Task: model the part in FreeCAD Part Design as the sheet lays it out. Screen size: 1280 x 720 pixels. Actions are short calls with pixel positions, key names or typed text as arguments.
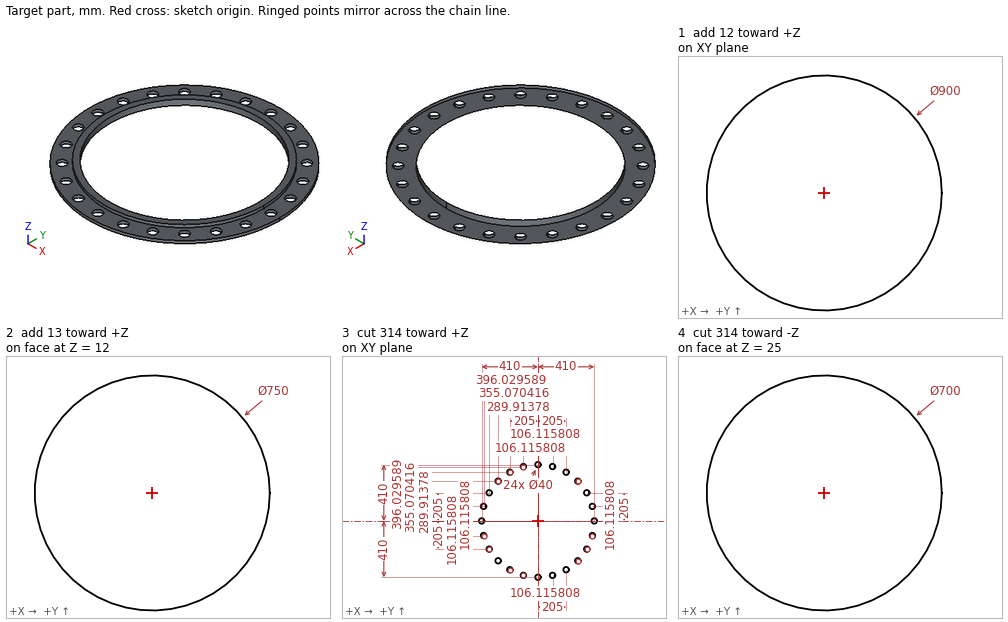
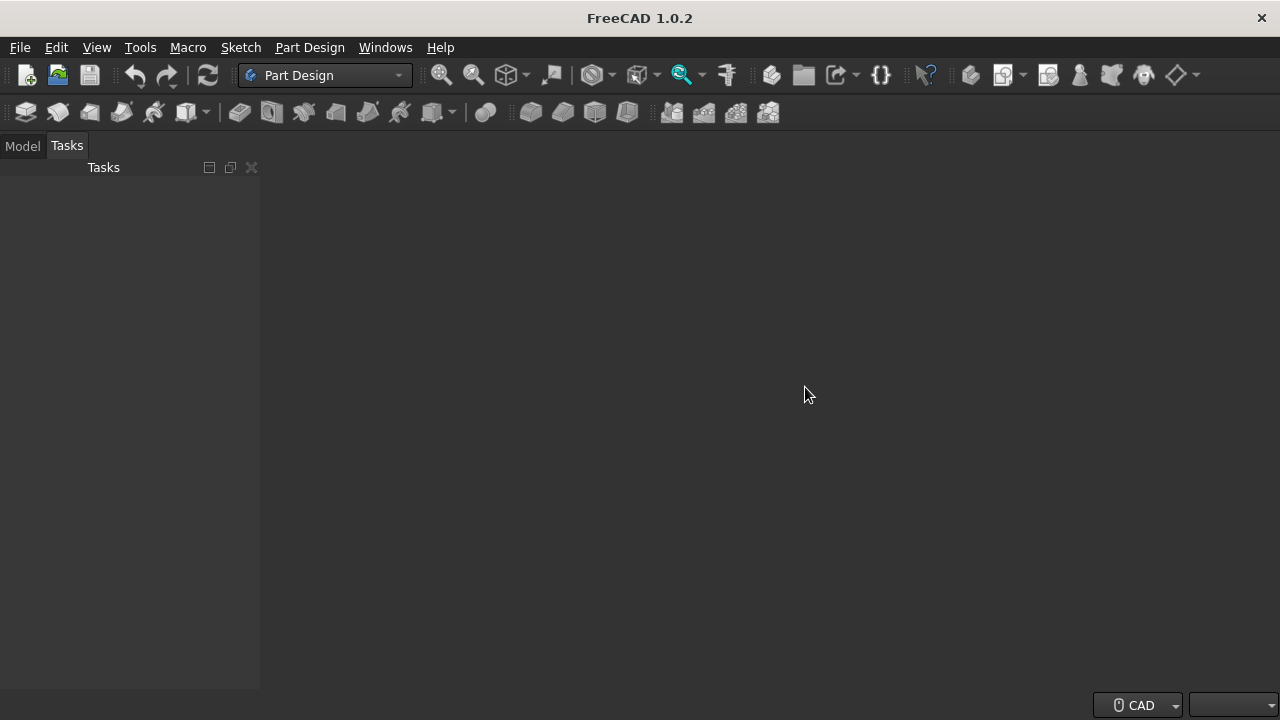
click(26, 76)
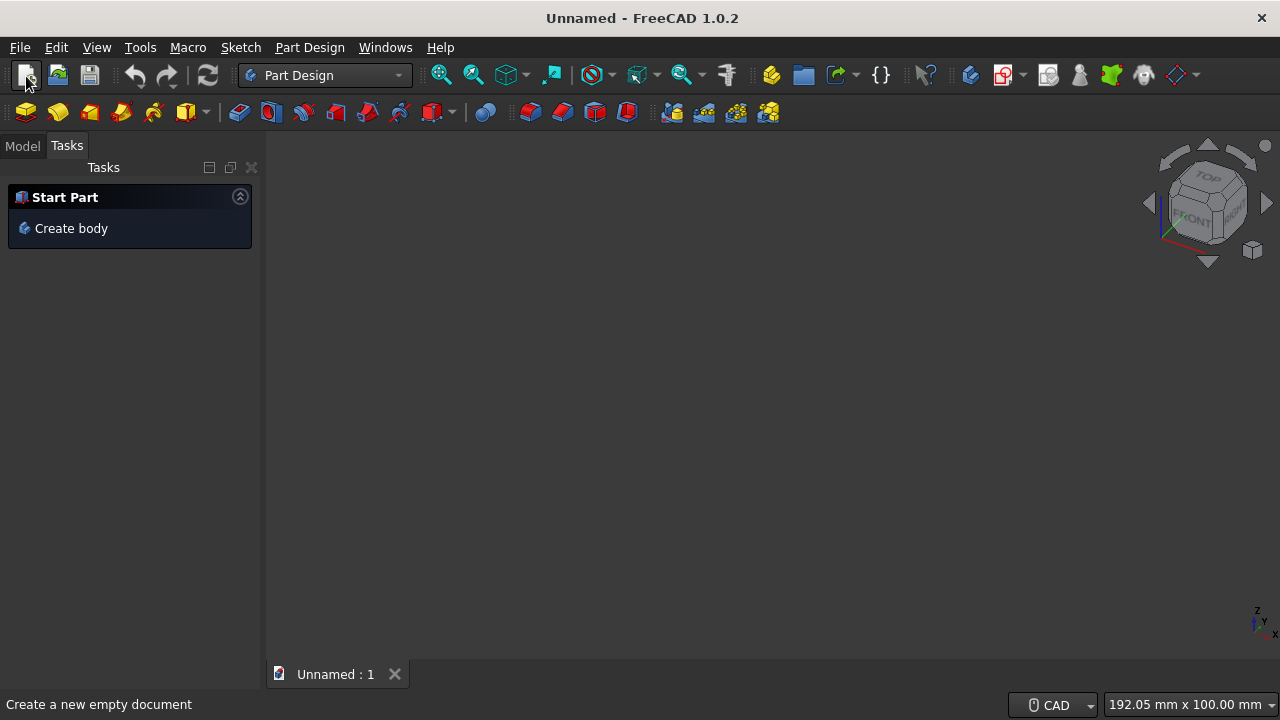
click(1004, 76)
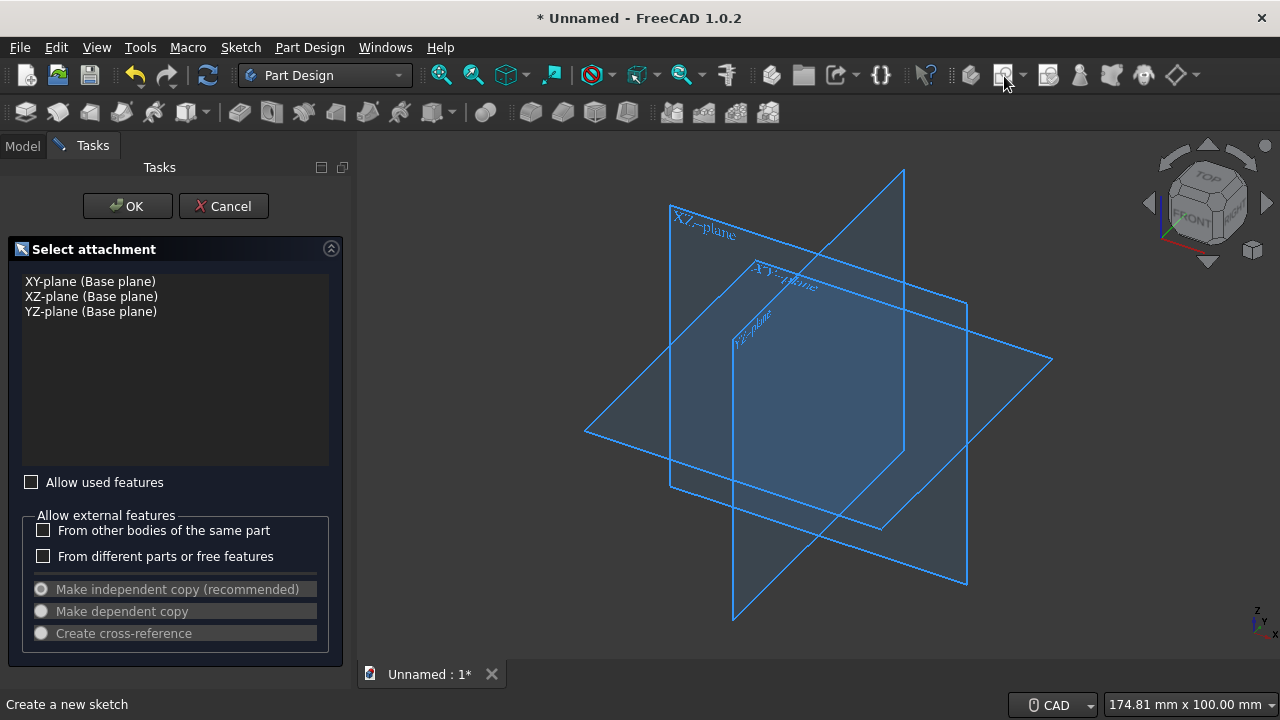
click(82, 282)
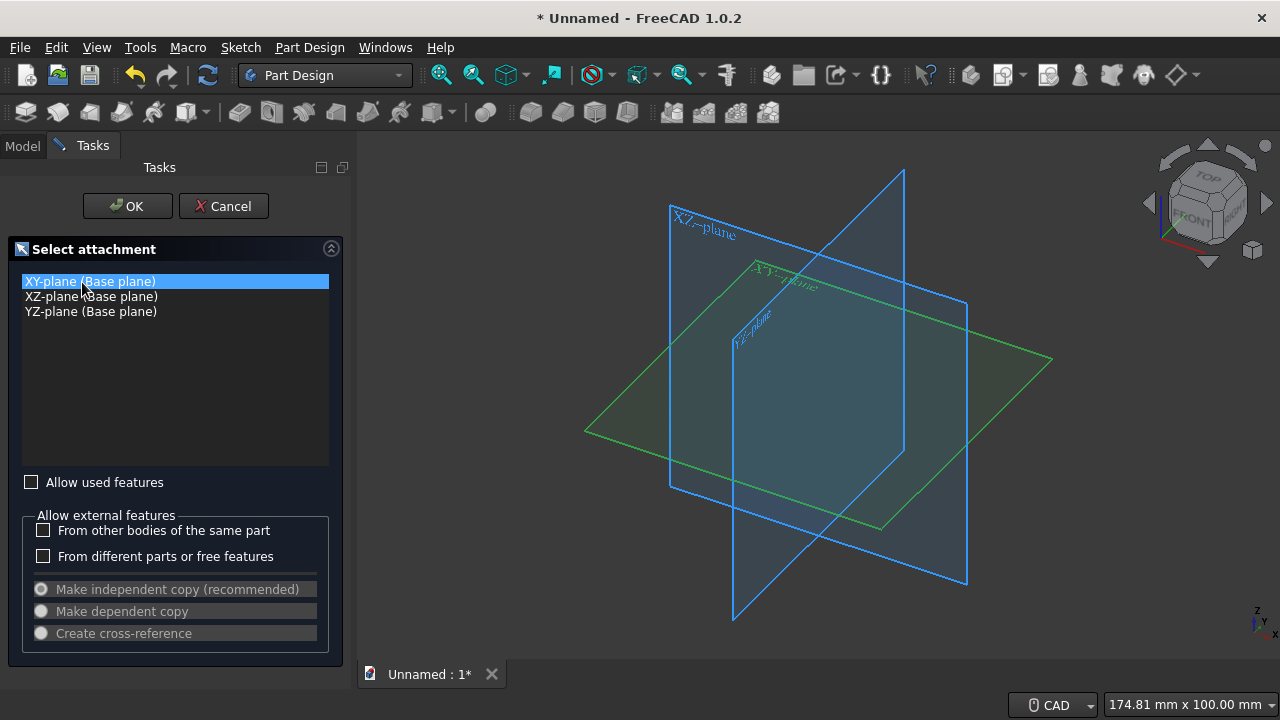
click(128, 206)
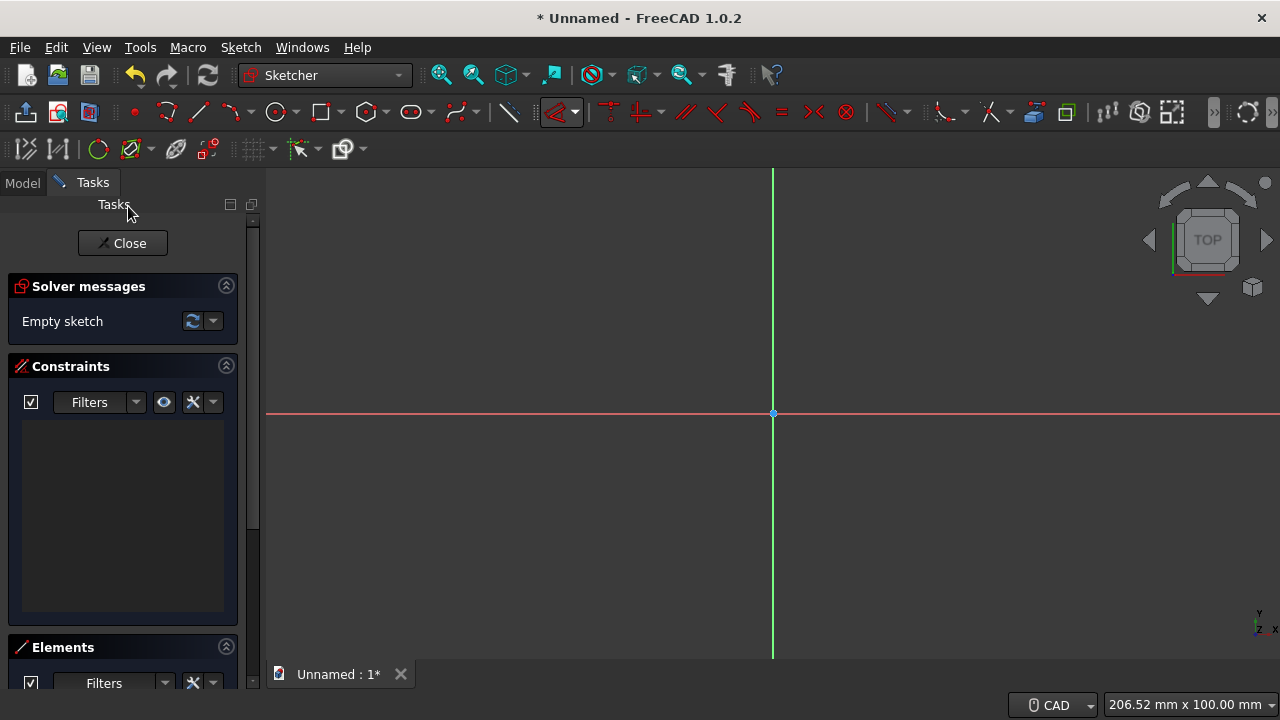
scroll(699, 414, down, 13)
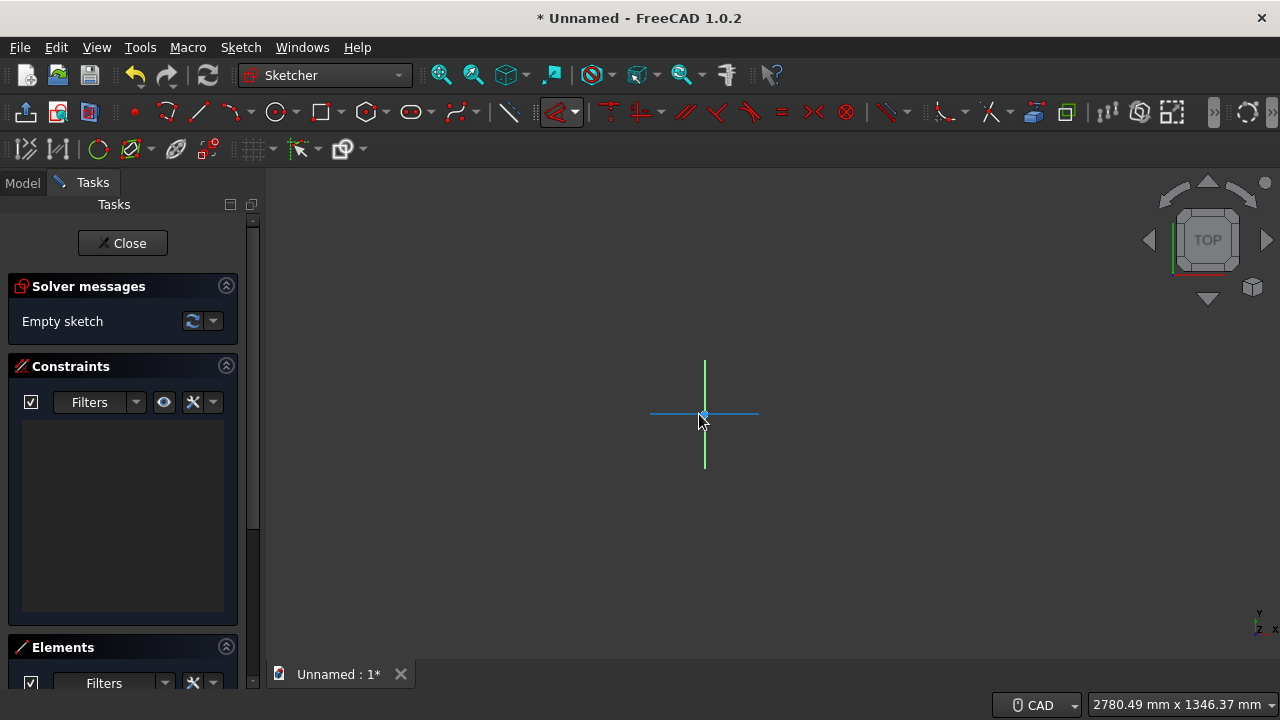
click(276, 112)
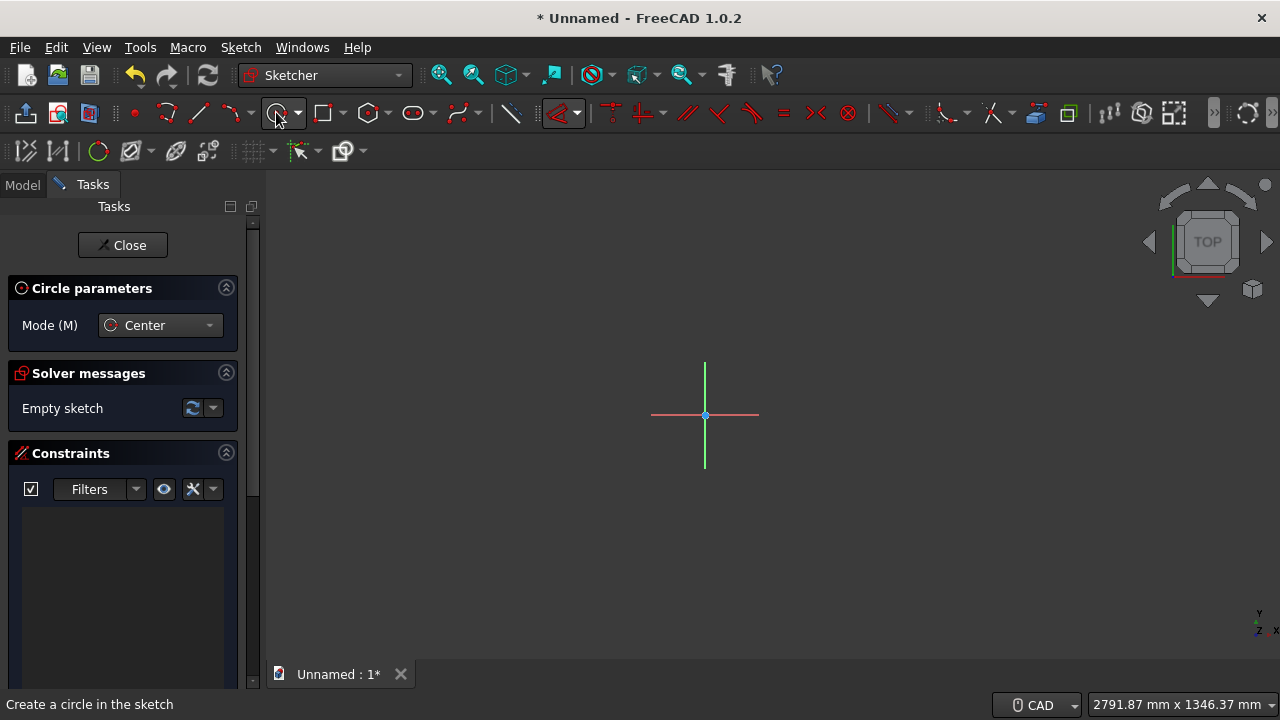
click(705, 415)
click(821, 300)
key(Escape)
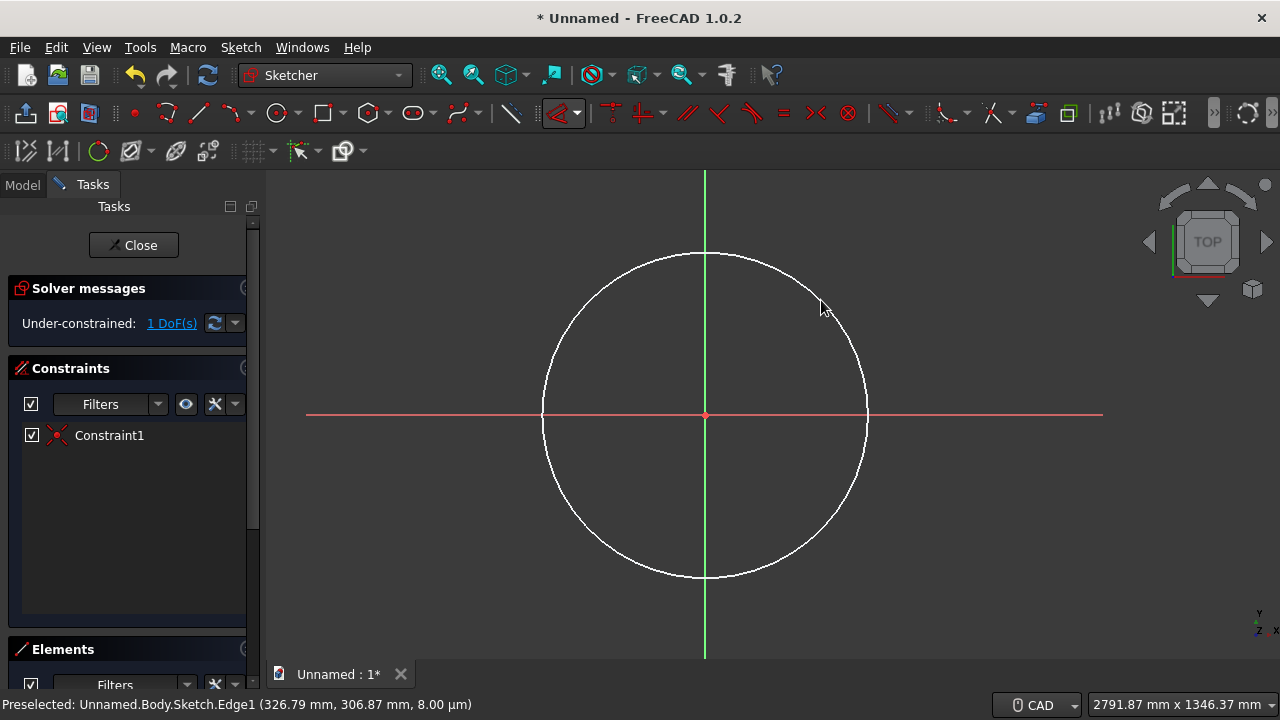
click(558, 114)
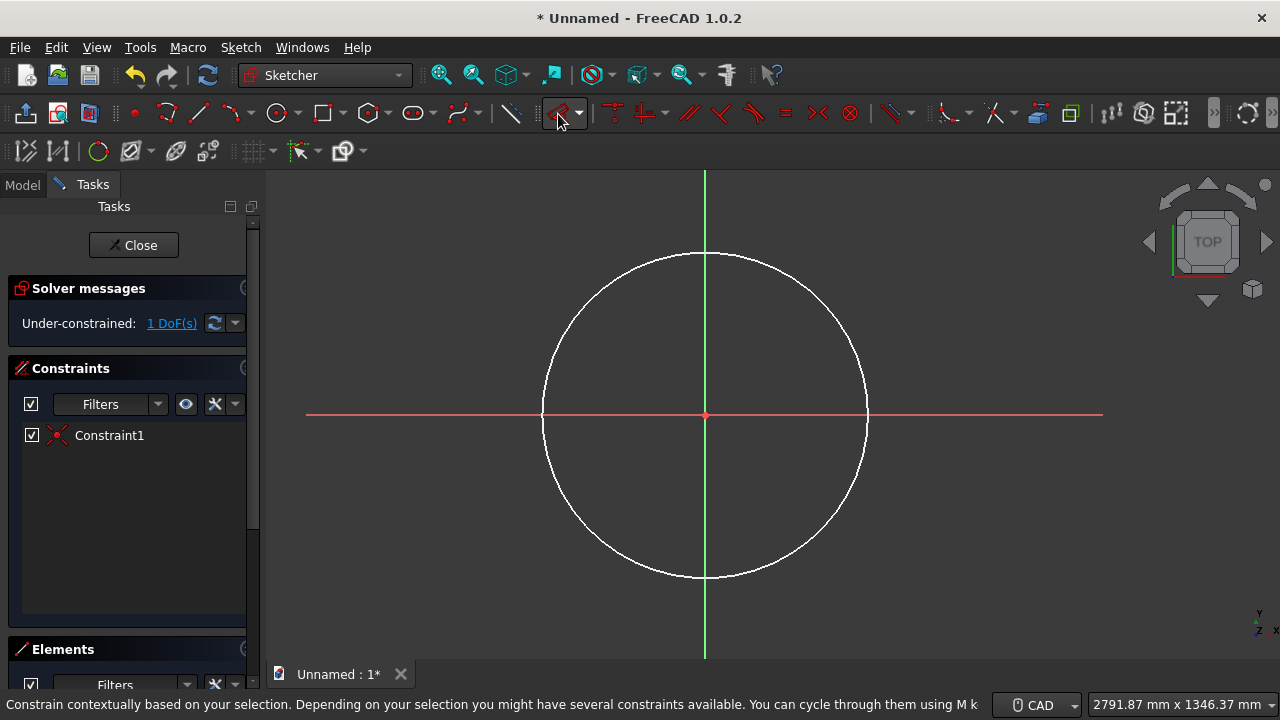
click(820, 300)
click(843, 277)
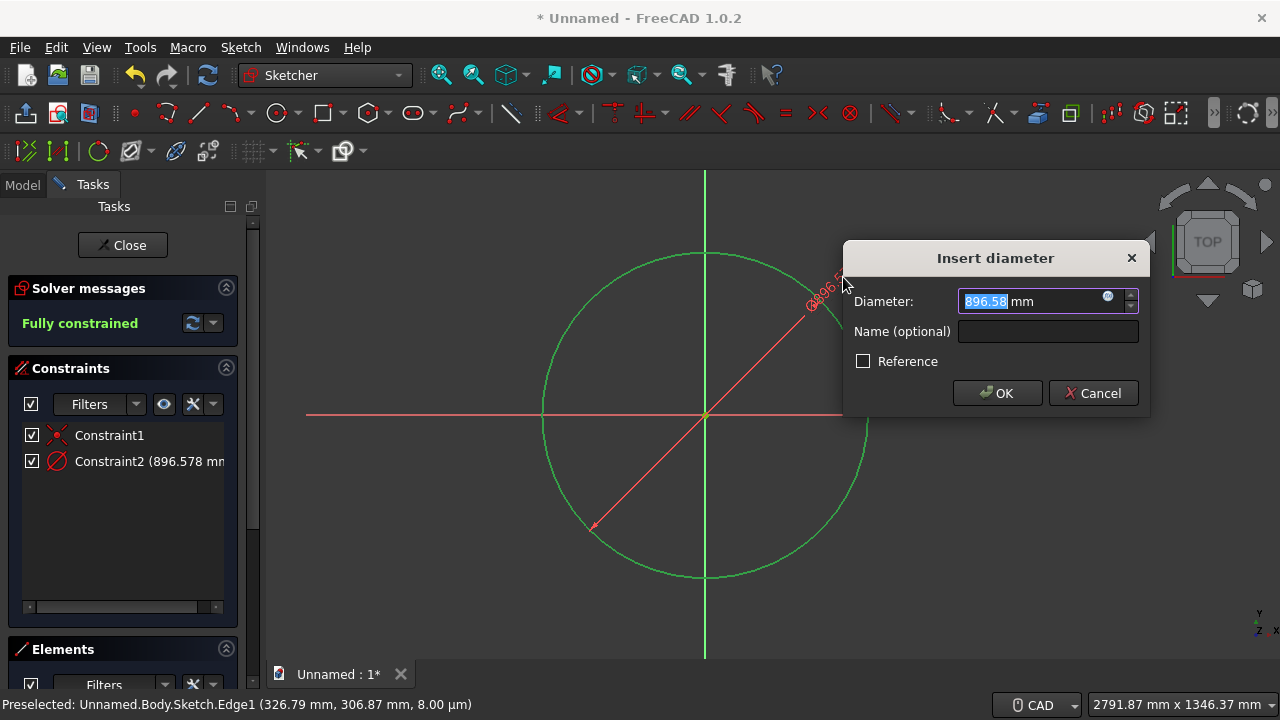
text(900)
key(Return)
key(Escape)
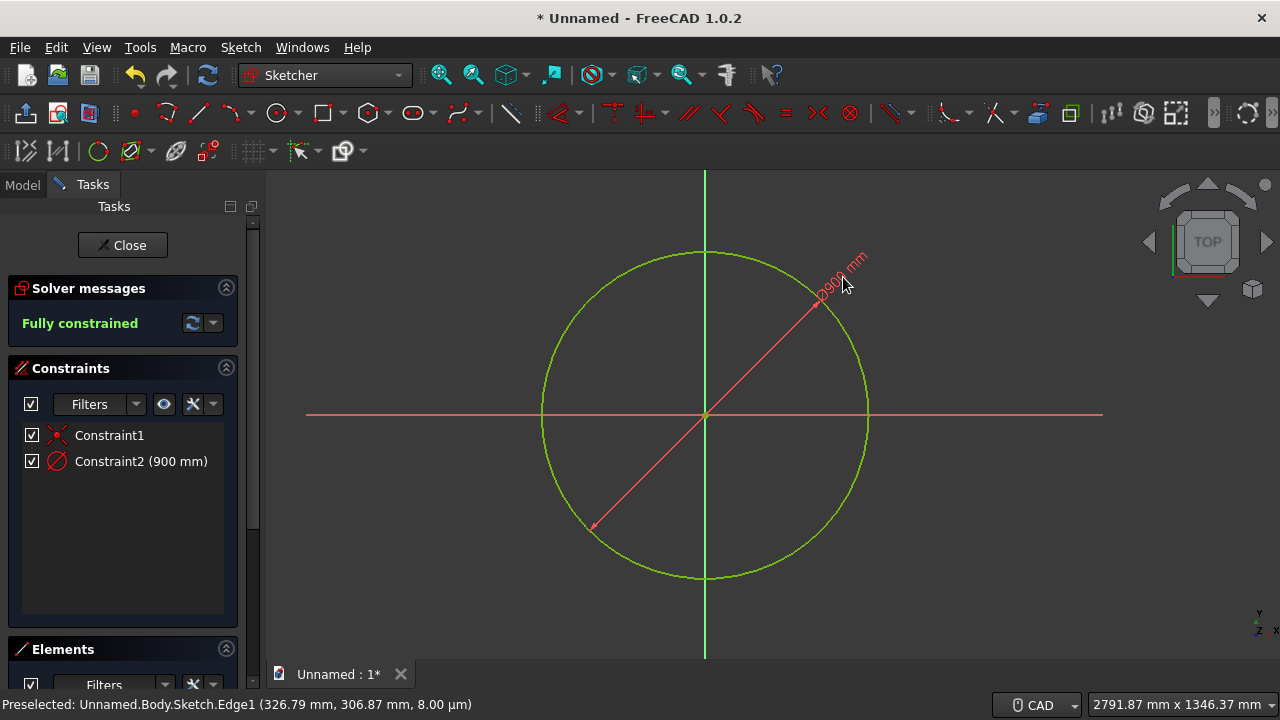
click(123, 245)